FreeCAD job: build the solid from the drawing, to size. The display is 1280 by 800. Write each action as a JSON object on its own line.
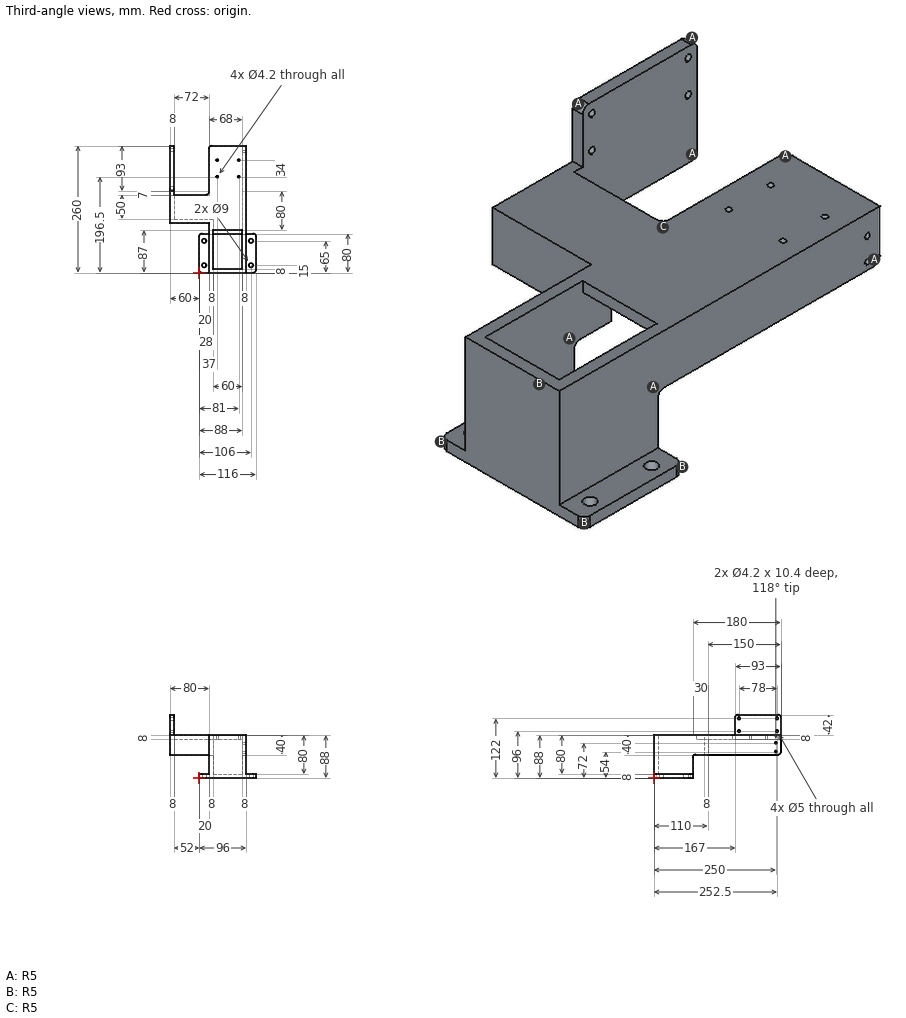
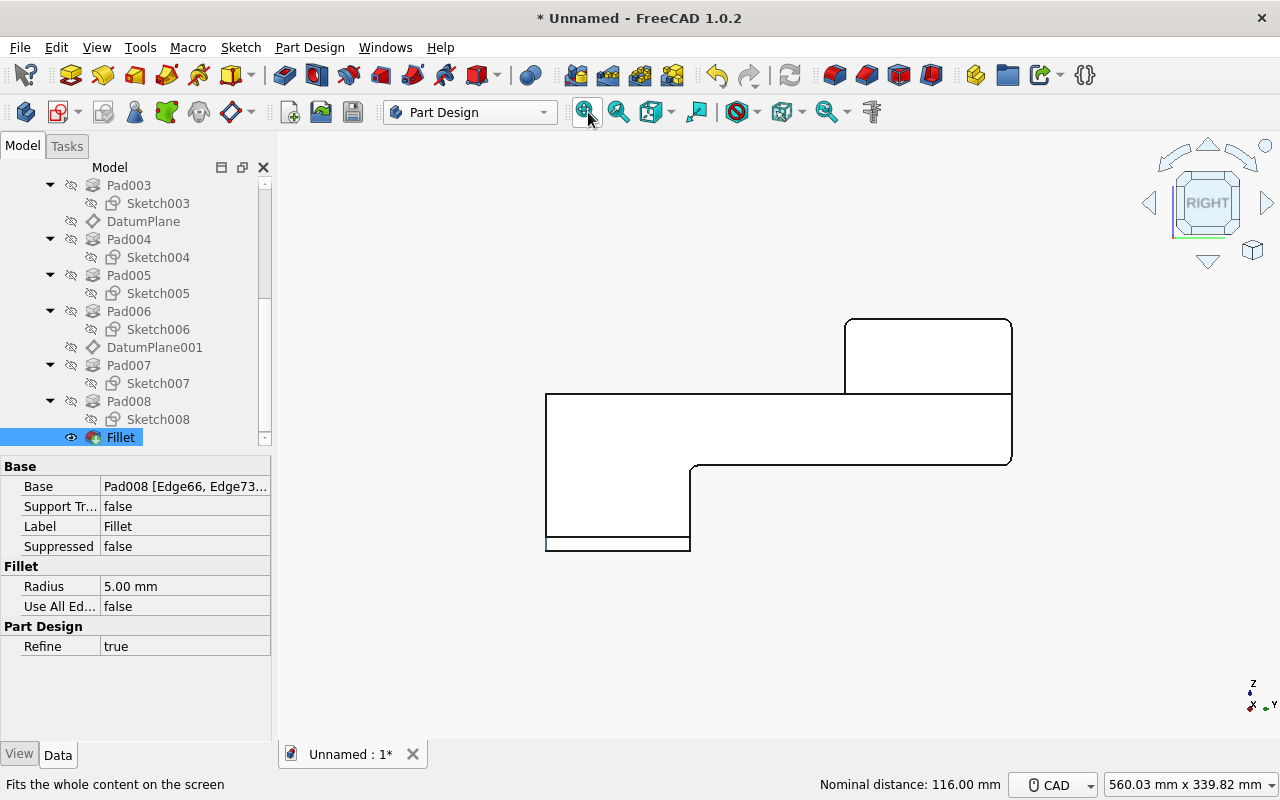
{"action": "left_click", "coordinate": [690, 543], "text": "ctrl"}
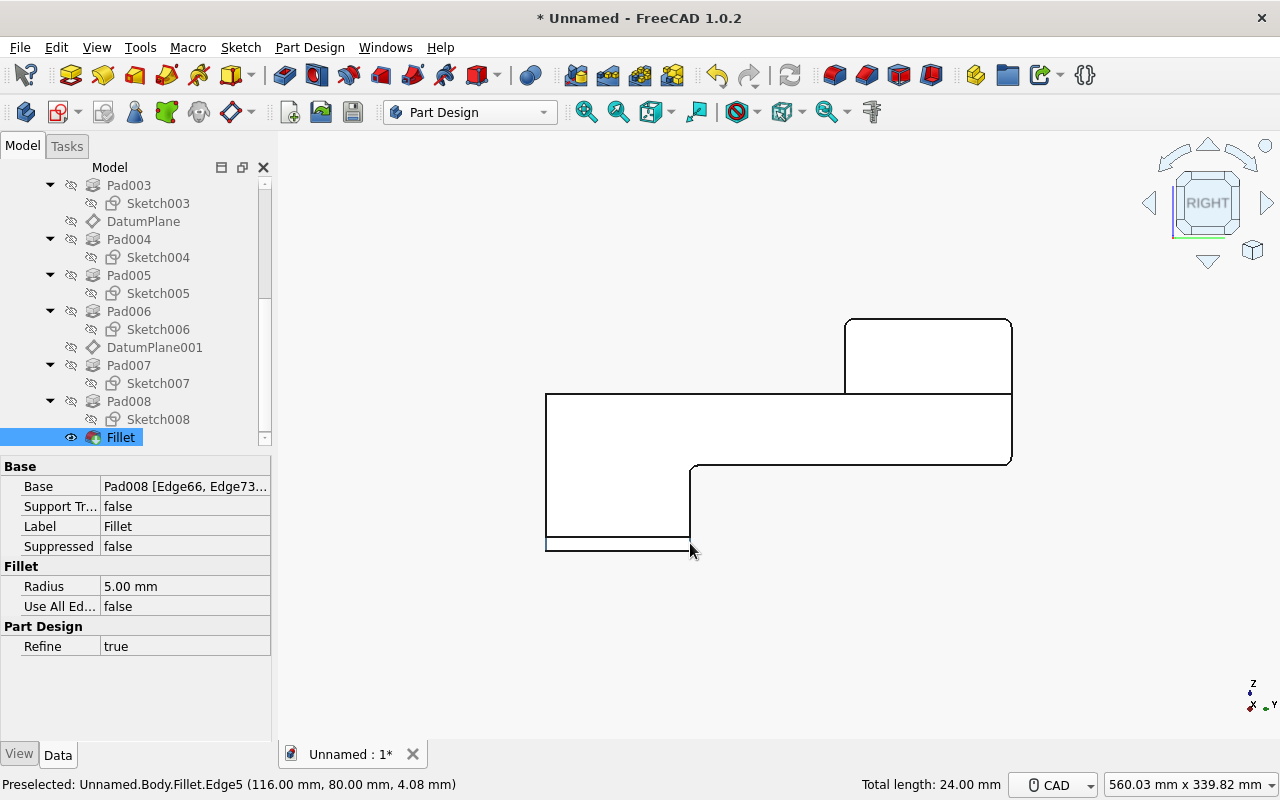
{"action": "scroll", "coordinate": [690, 543], "scroll_direction": "up", "scroll_amount": 6}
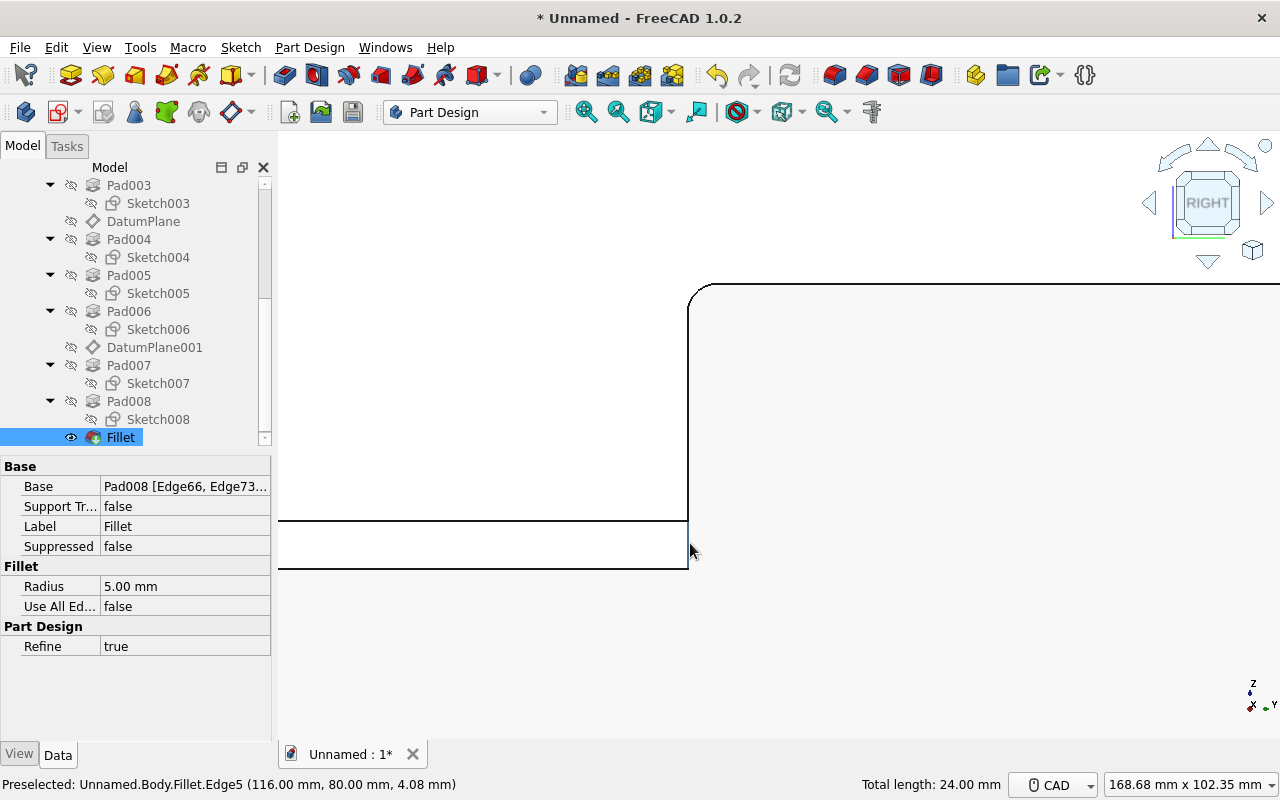
{"action": "left_click", "coordinate": [588, 112]}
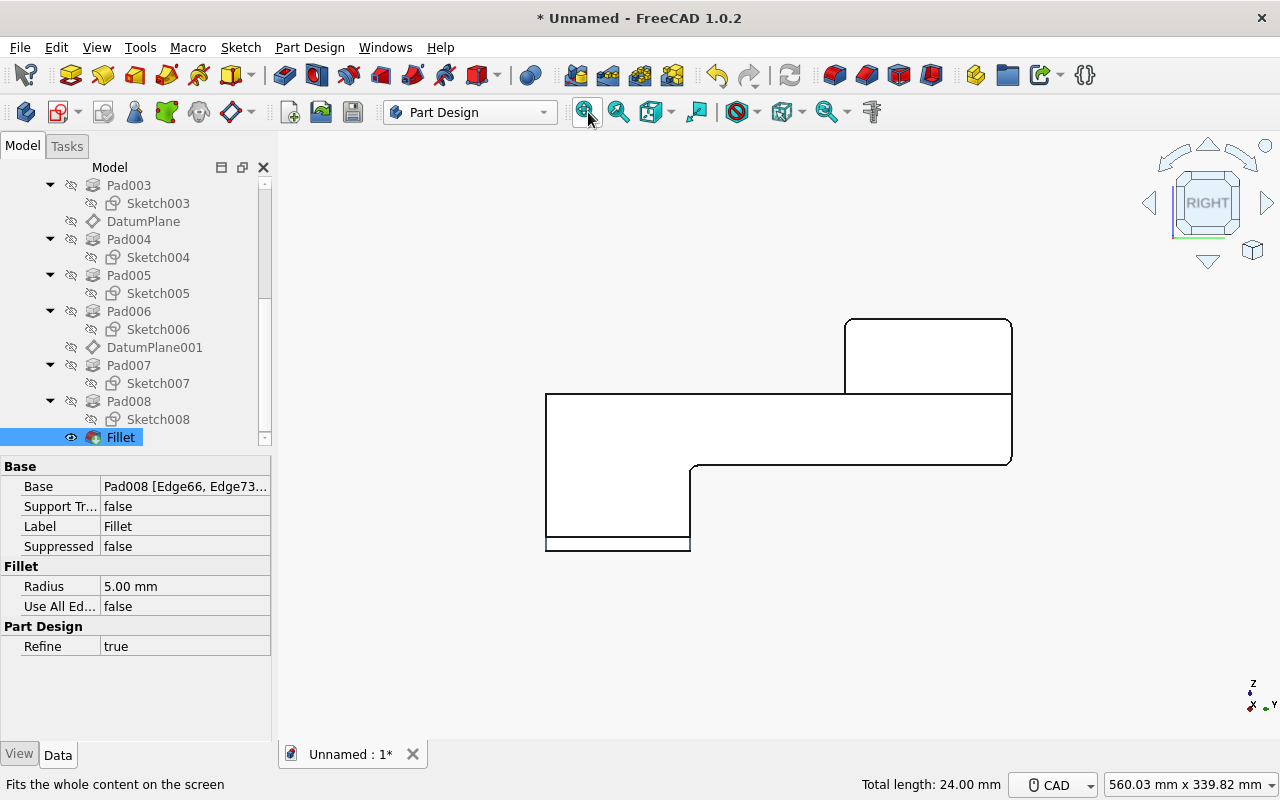
{"action": "key", "text": "5"}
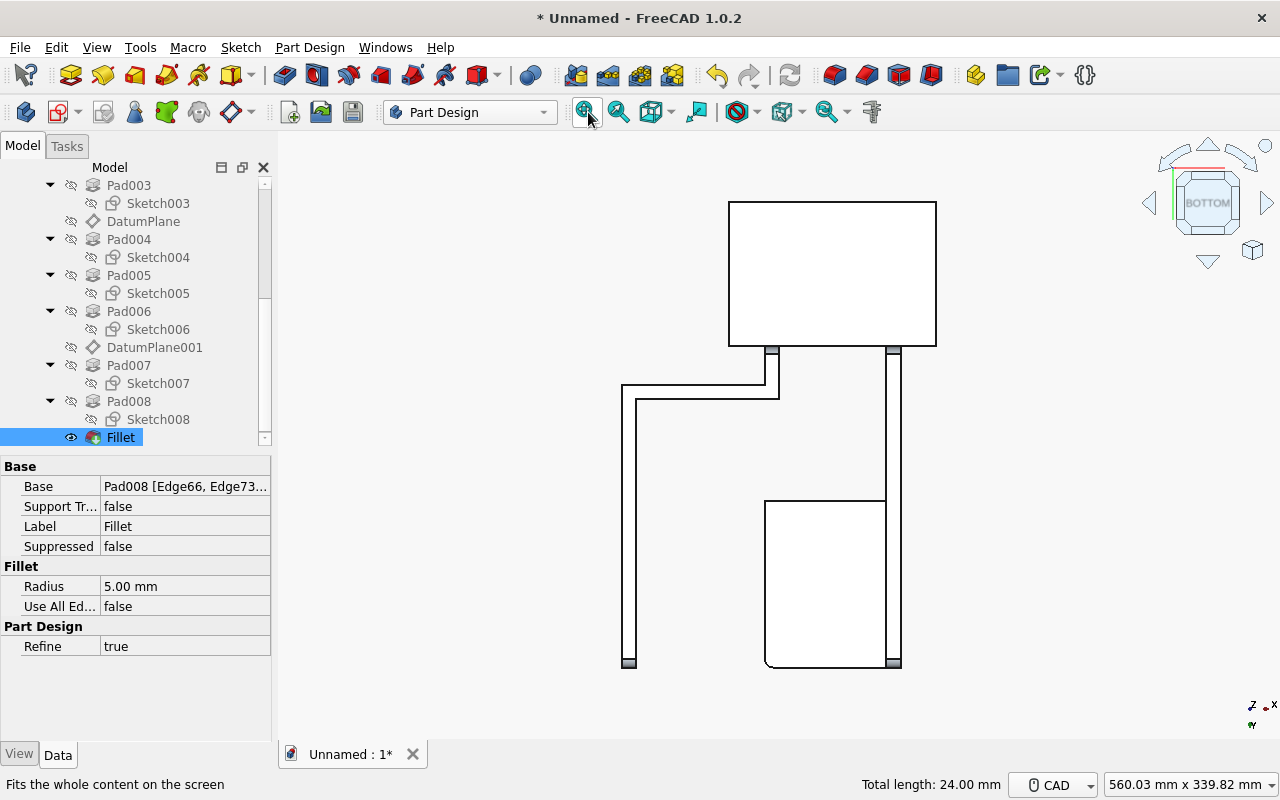
{"action": "scroll", "coordinate": [729, 345], "scroll_direction": "up", "scroll_amount": 6}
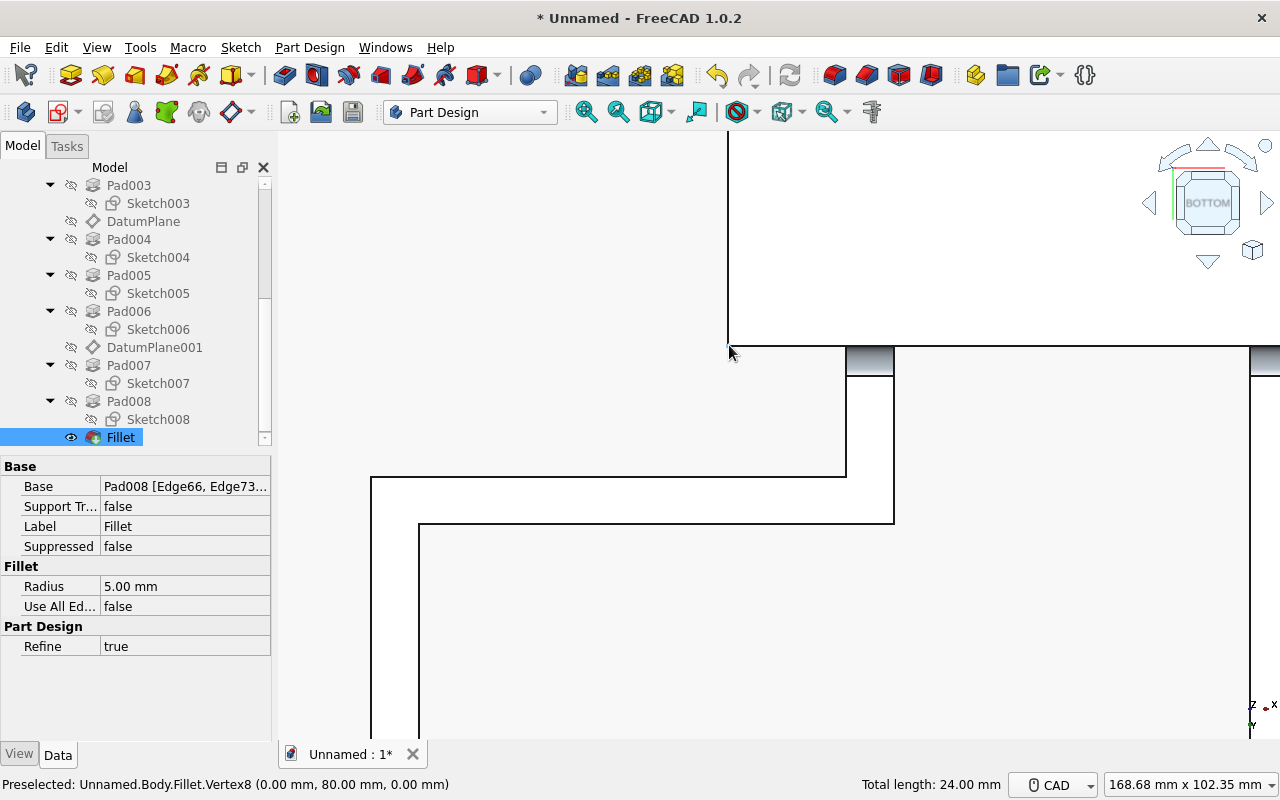
{"action": "left_click", "coordinate": [588, 112]}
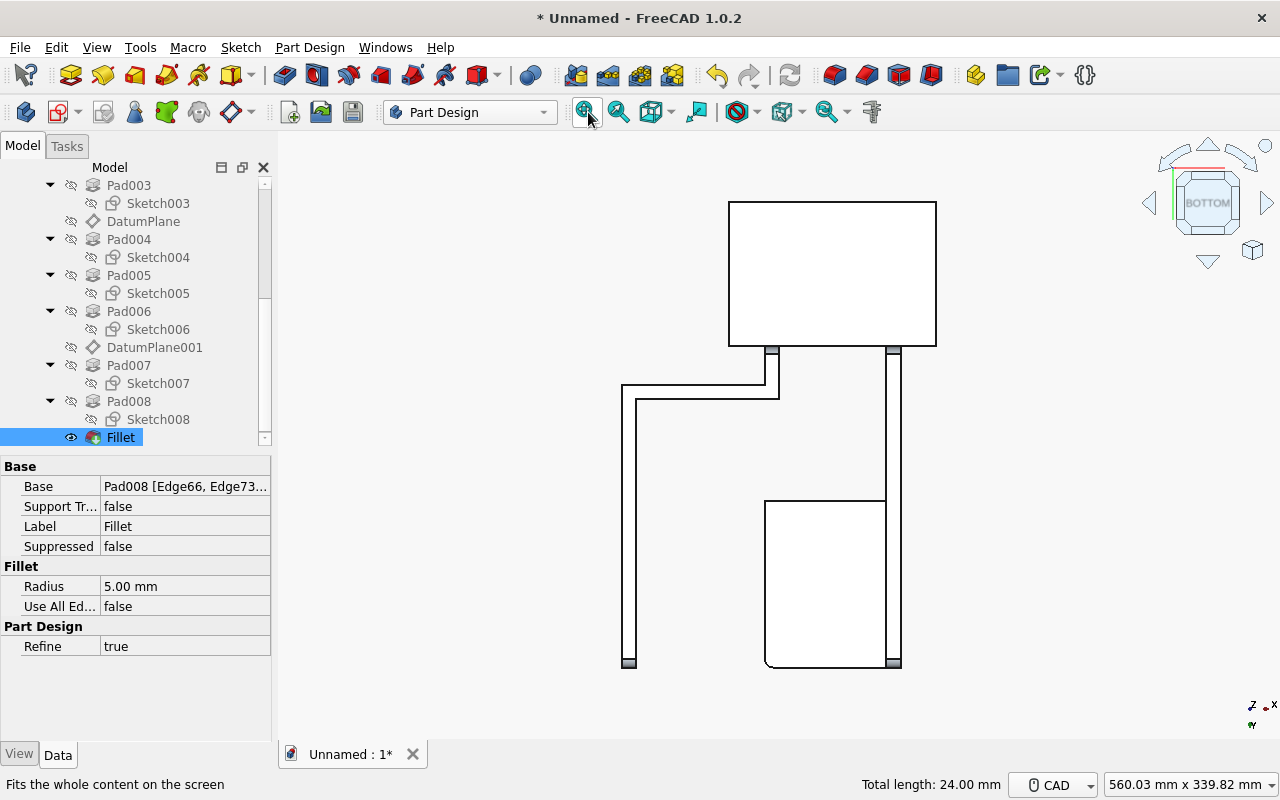
{"action": "key", "text": "4"}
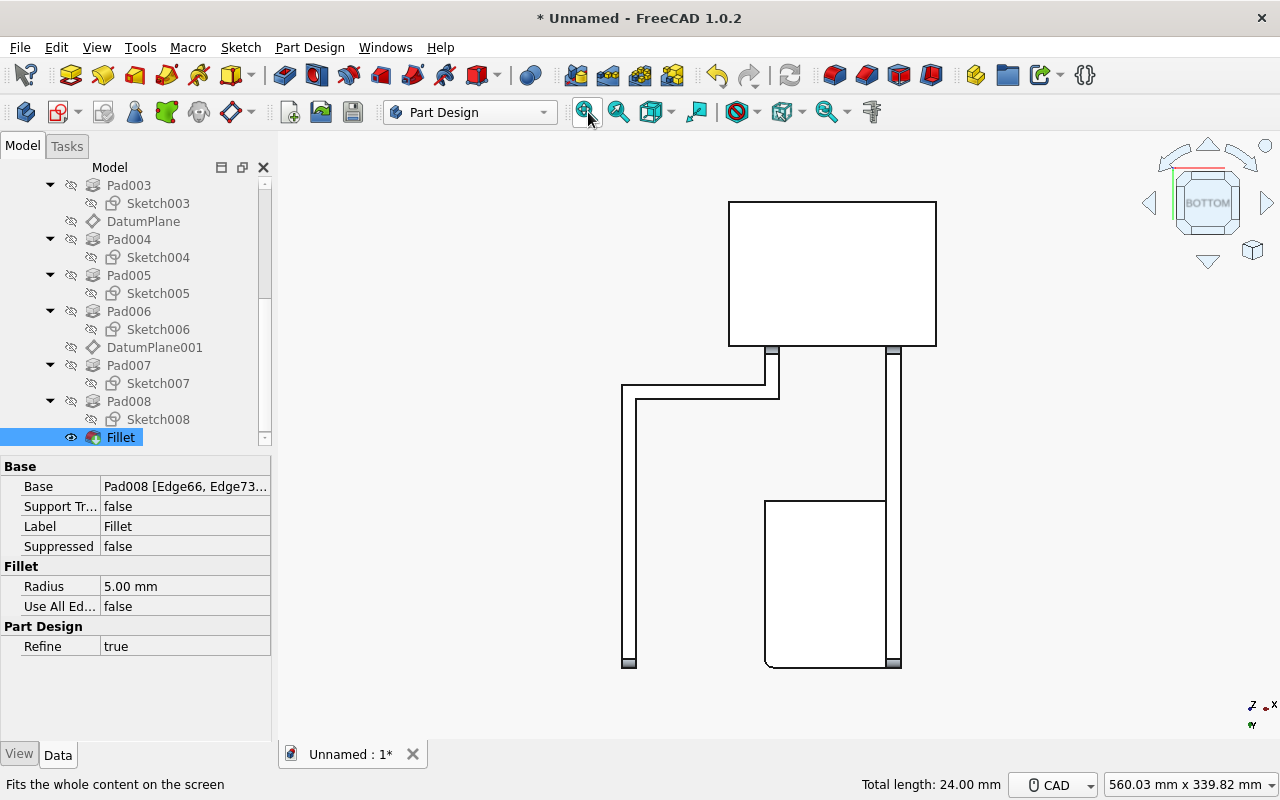
{"action": "left_click", "coordinate": [588, 112]}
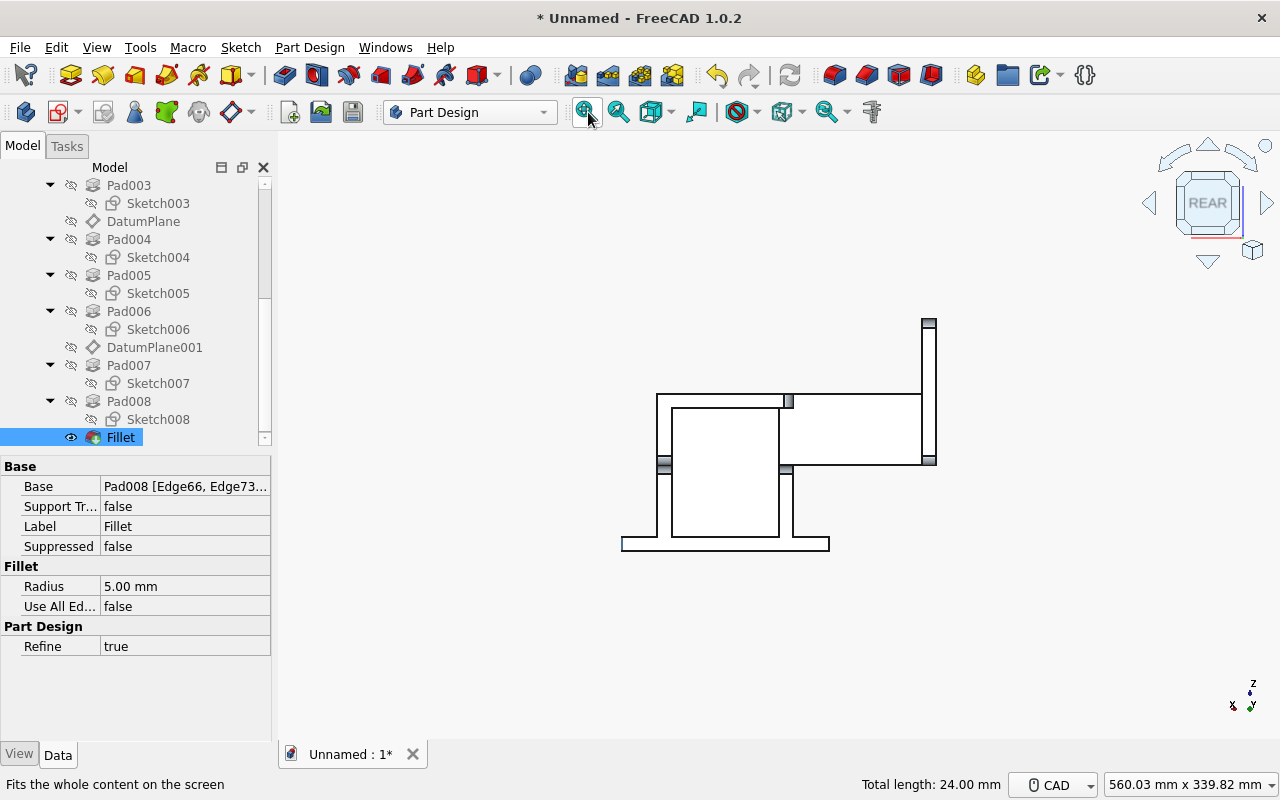
{"action": "left_click", "coordinate": [829, 543], "text": "ctrl"}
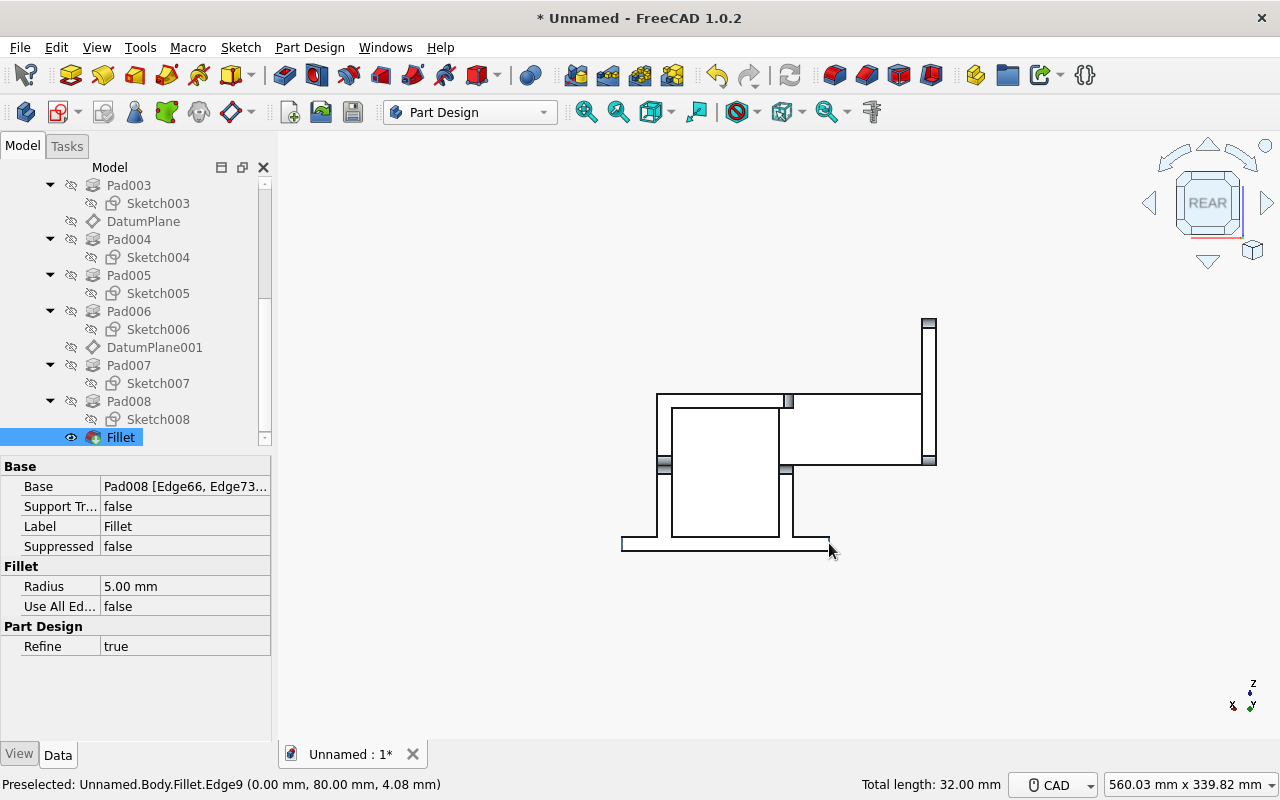
{"action": "left_click", "coordinate": [836, 76]}